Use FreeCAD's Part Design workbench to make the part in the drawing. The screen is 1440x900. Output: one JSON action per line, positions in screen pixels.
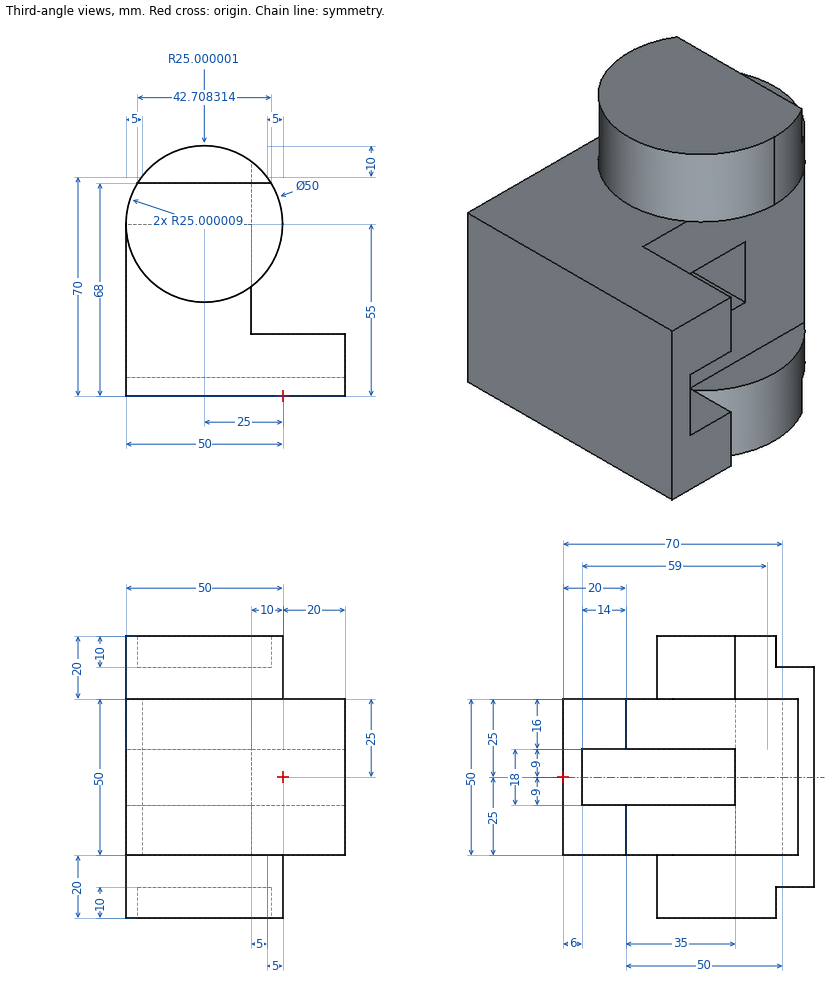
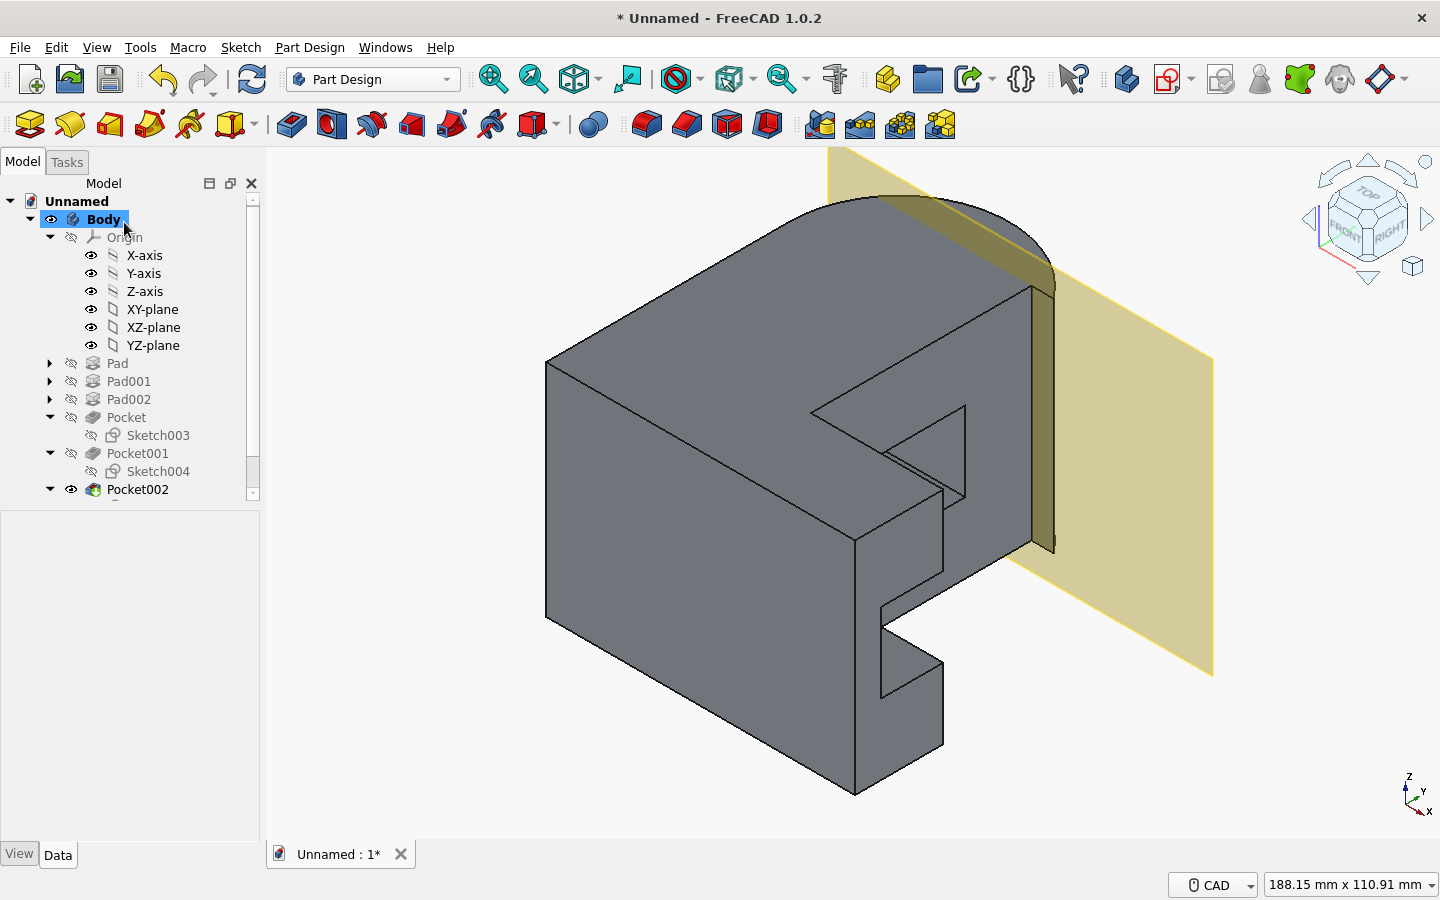
{"action": "scroll", "coordinate": [100, 341], "scroll_direction": "down", "scroll_amount": 3}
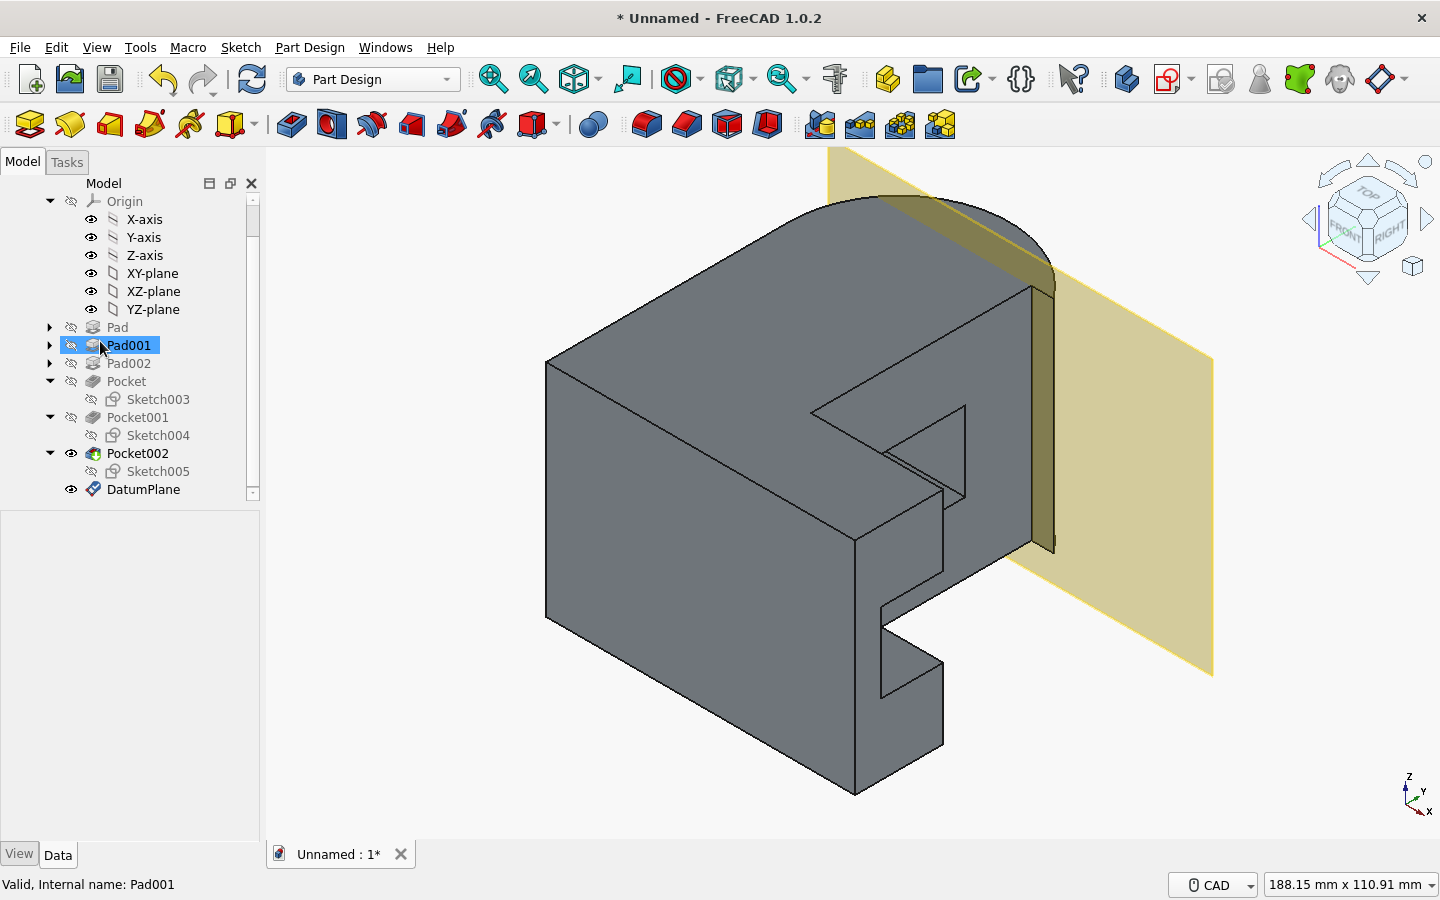
{"action": "left_click", "coordinate": [116, 489]}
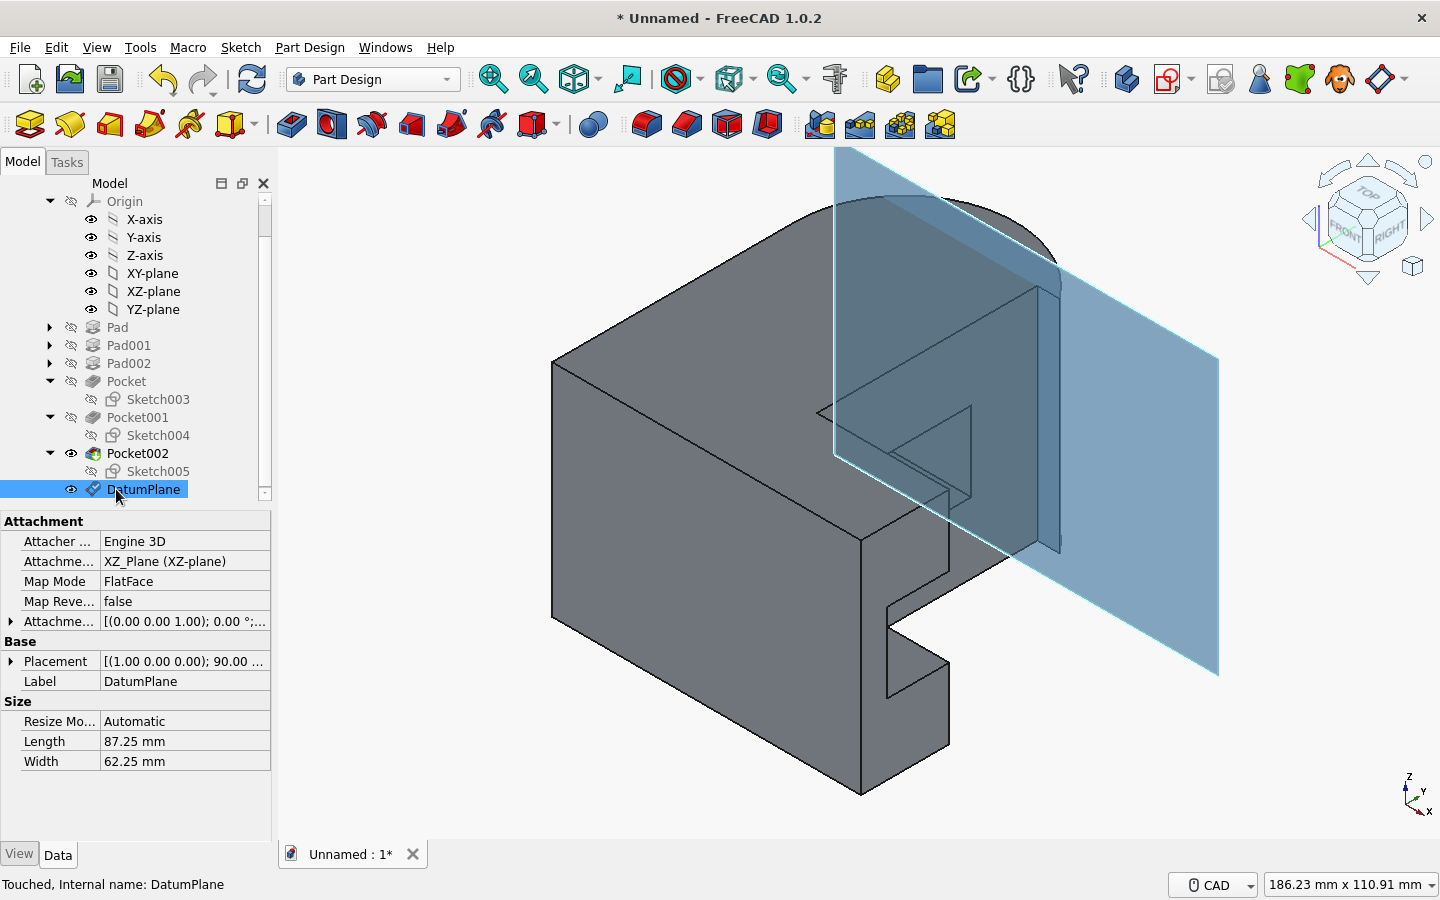
{"action": "left_click", "coordinate": [1168, 80]}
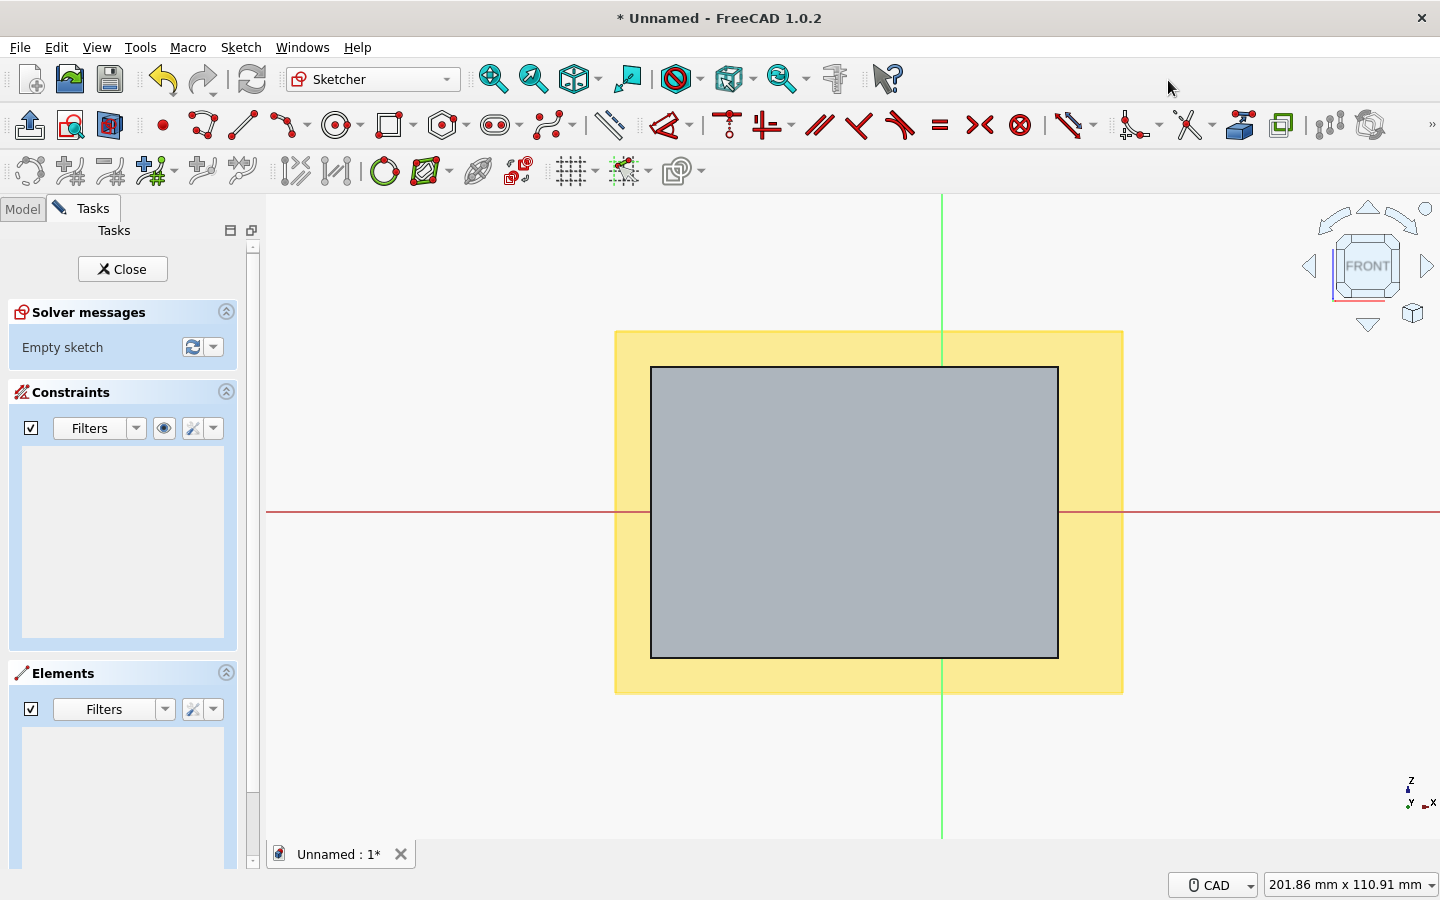
{"action": "left_click", "coordinate": [110, 126]}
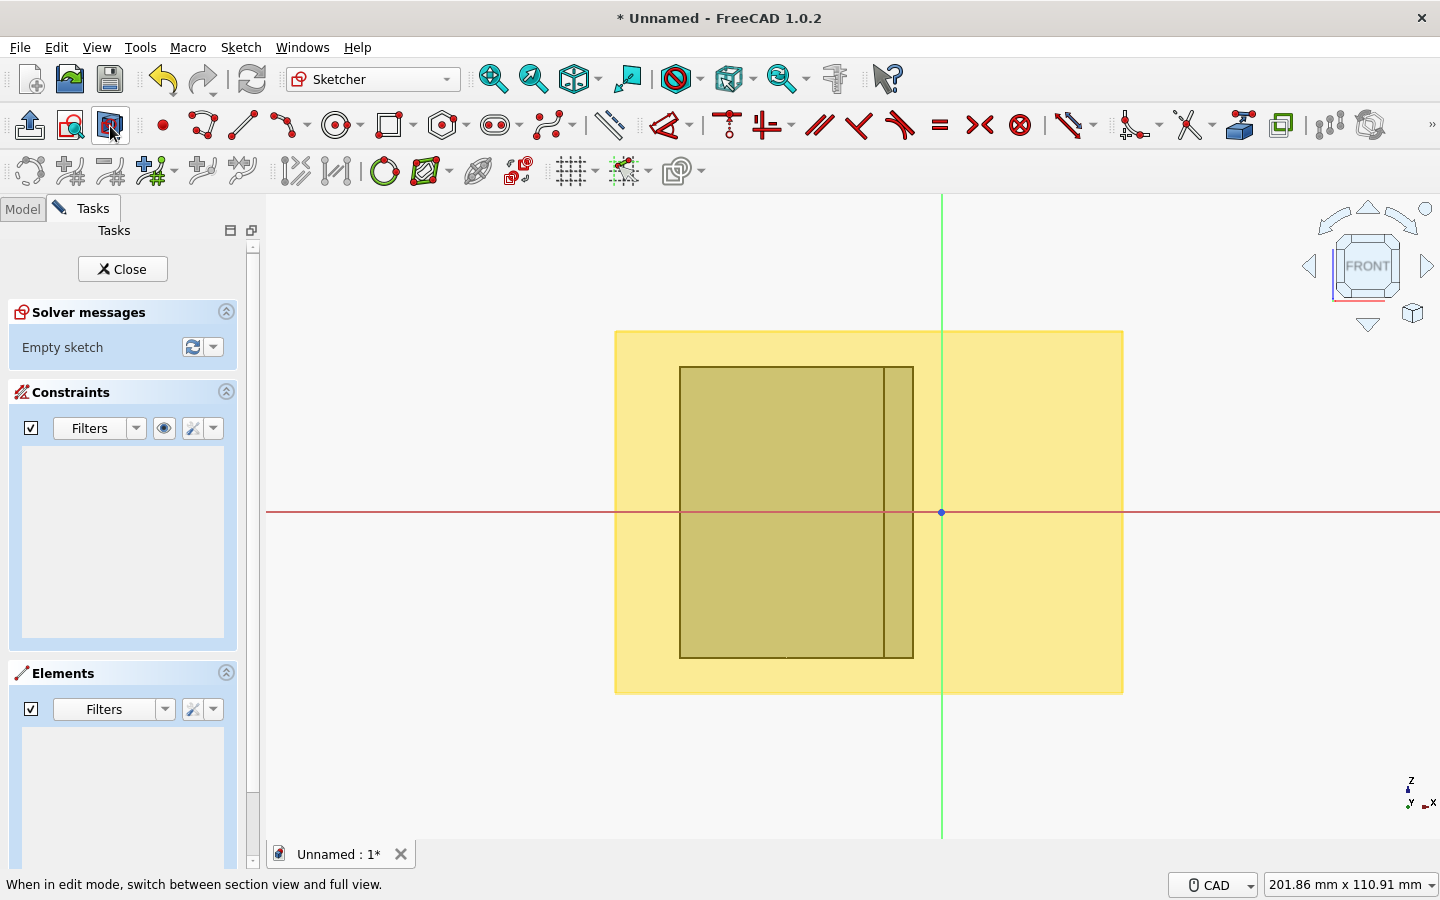
{"action": "scroll", "coordinate": [1174, 503], "scroll_direction": "up", "scroll_amount": 2}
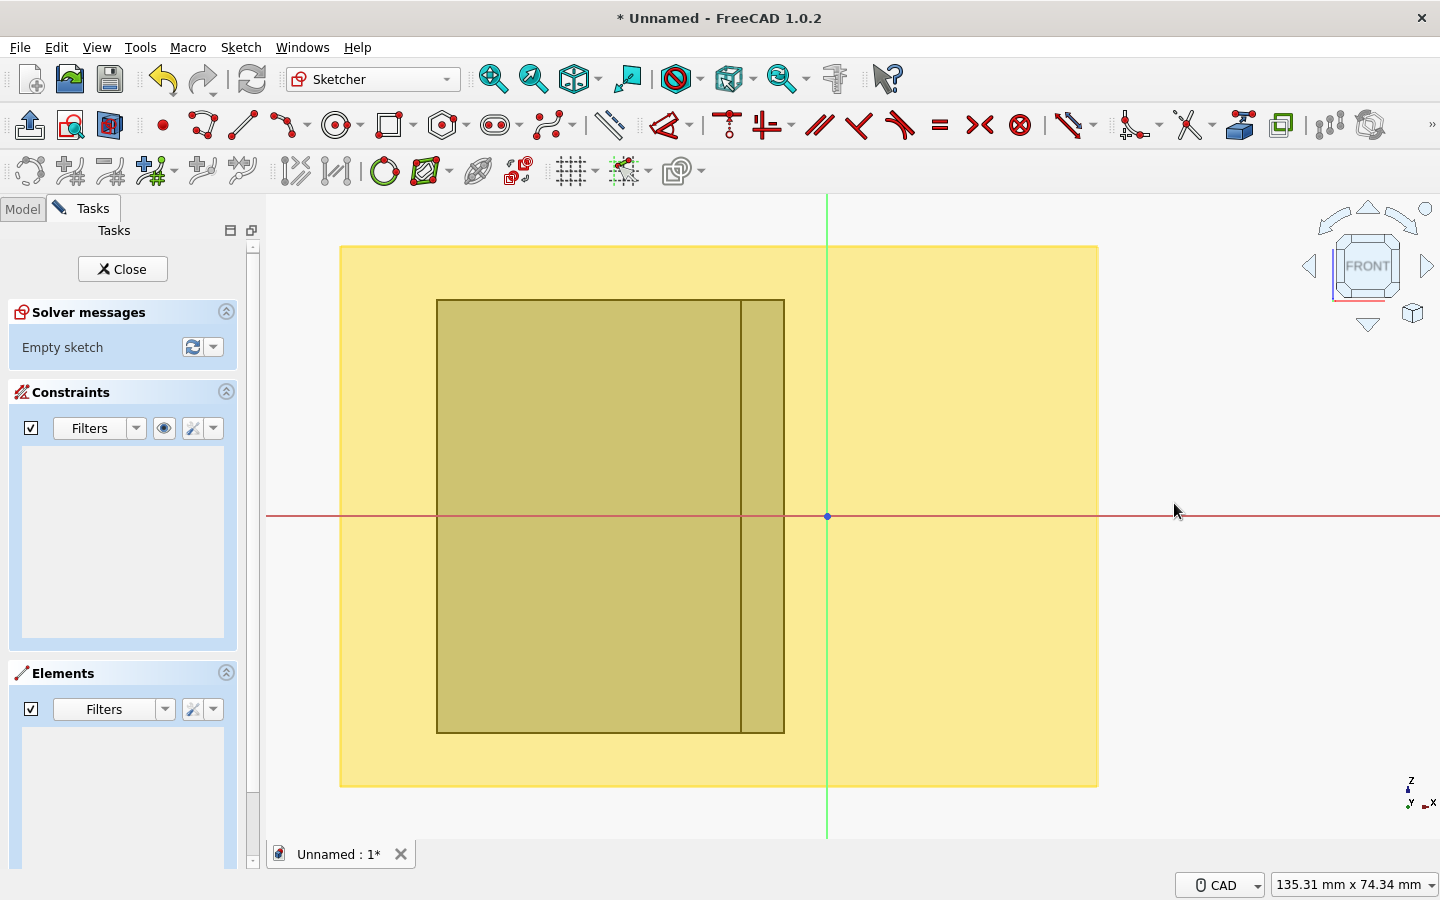
{"action": "key", "text": "g r"}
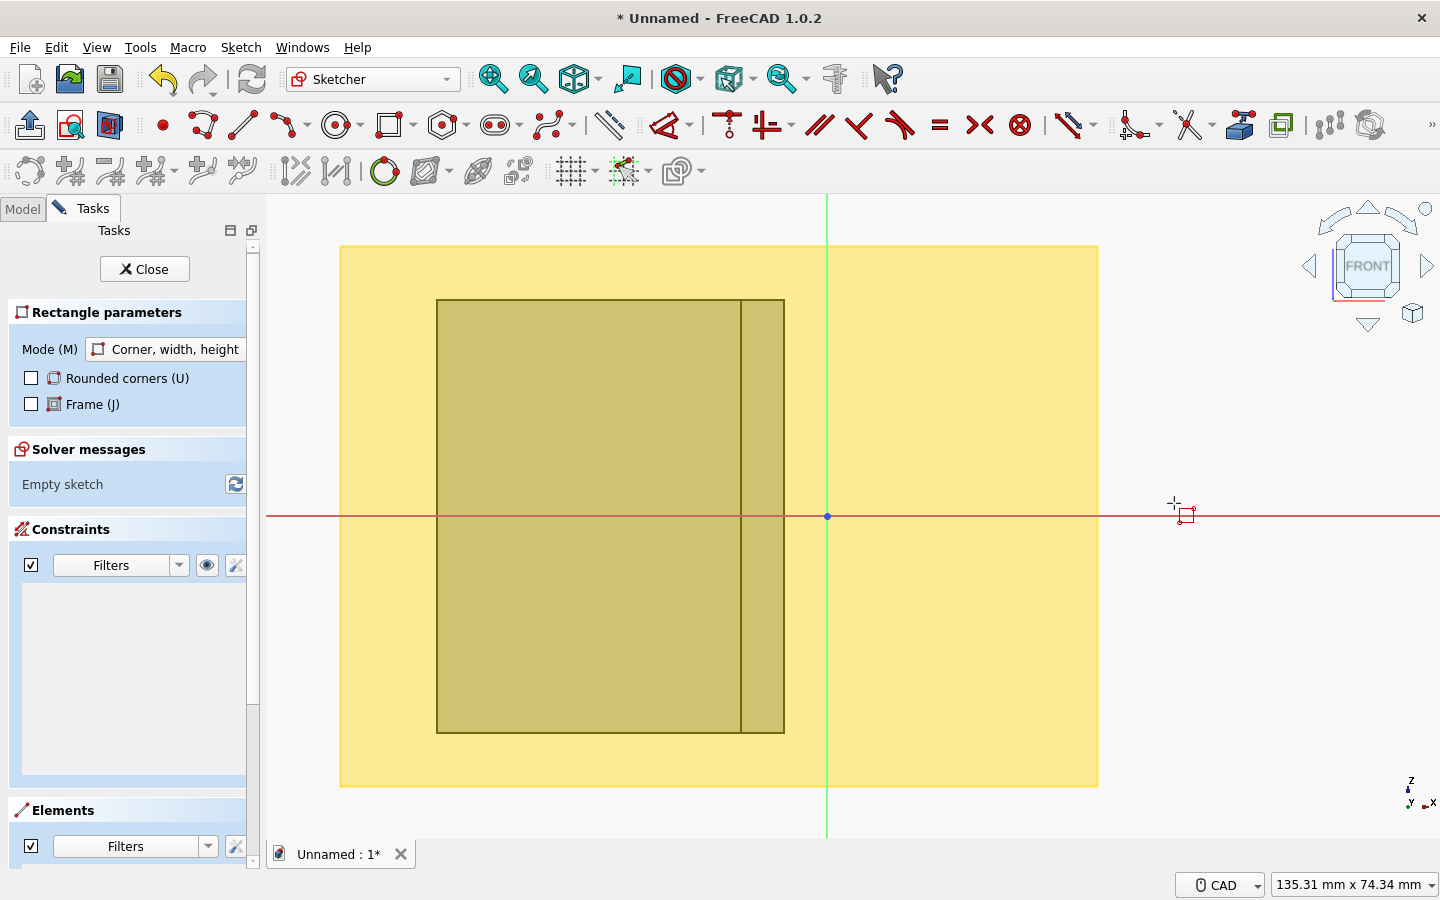
{"action": "left_click", "coordinate": [741, 300]}
{"action": "mouse_move", "coordinate": [784, 733]}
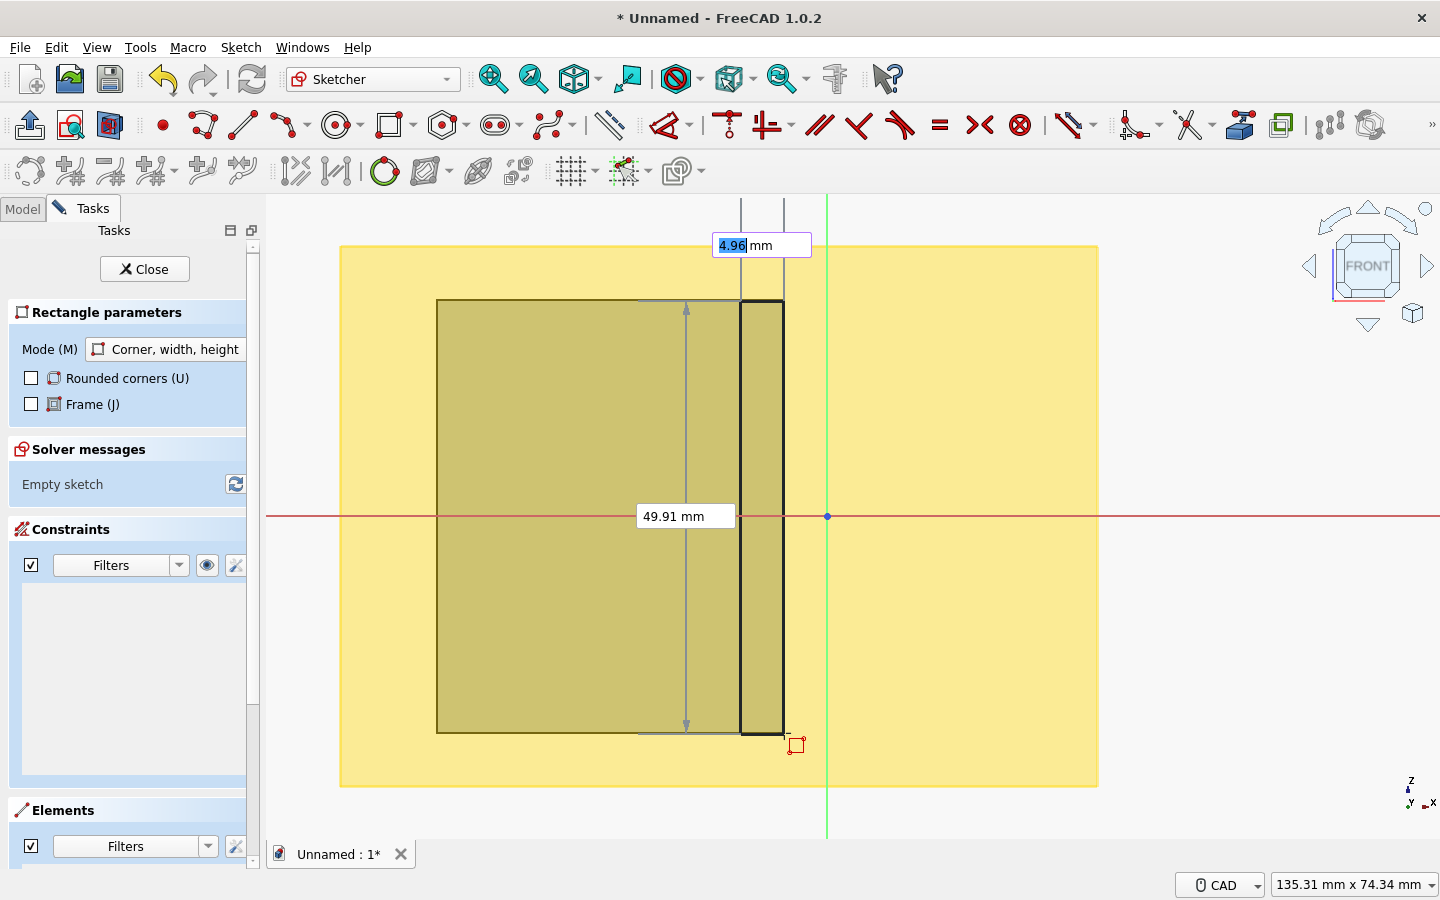
{"action": "type", "text": "5"}
{"action": "key", "text": "Tab"}
{"action": "type", "text": "50"}
{"action": "key", "text": "Return"}
{"action": "key", "text": "Escape"}